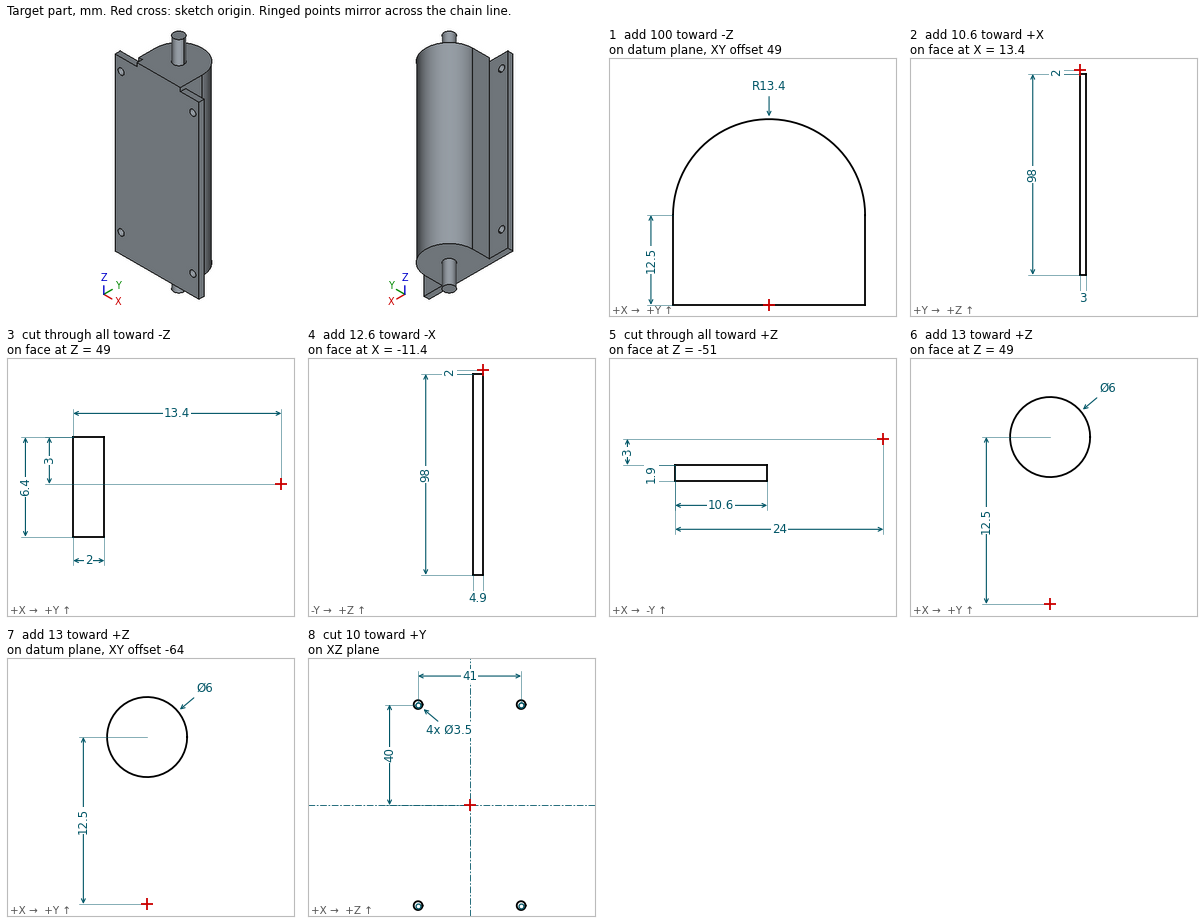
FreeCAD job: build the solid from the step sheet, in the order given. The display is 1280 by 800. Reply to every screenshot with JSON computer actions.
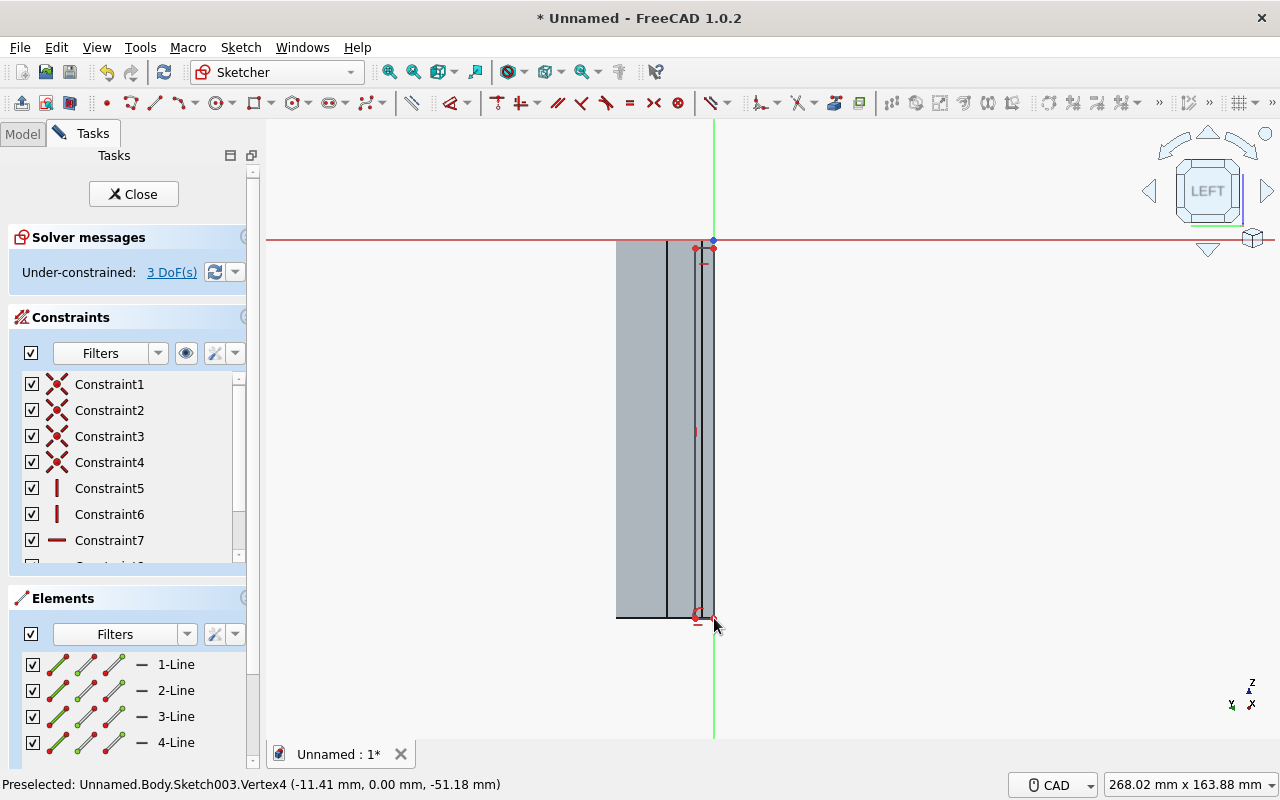
{"action": "left_click", "coordinate": [450, 104]}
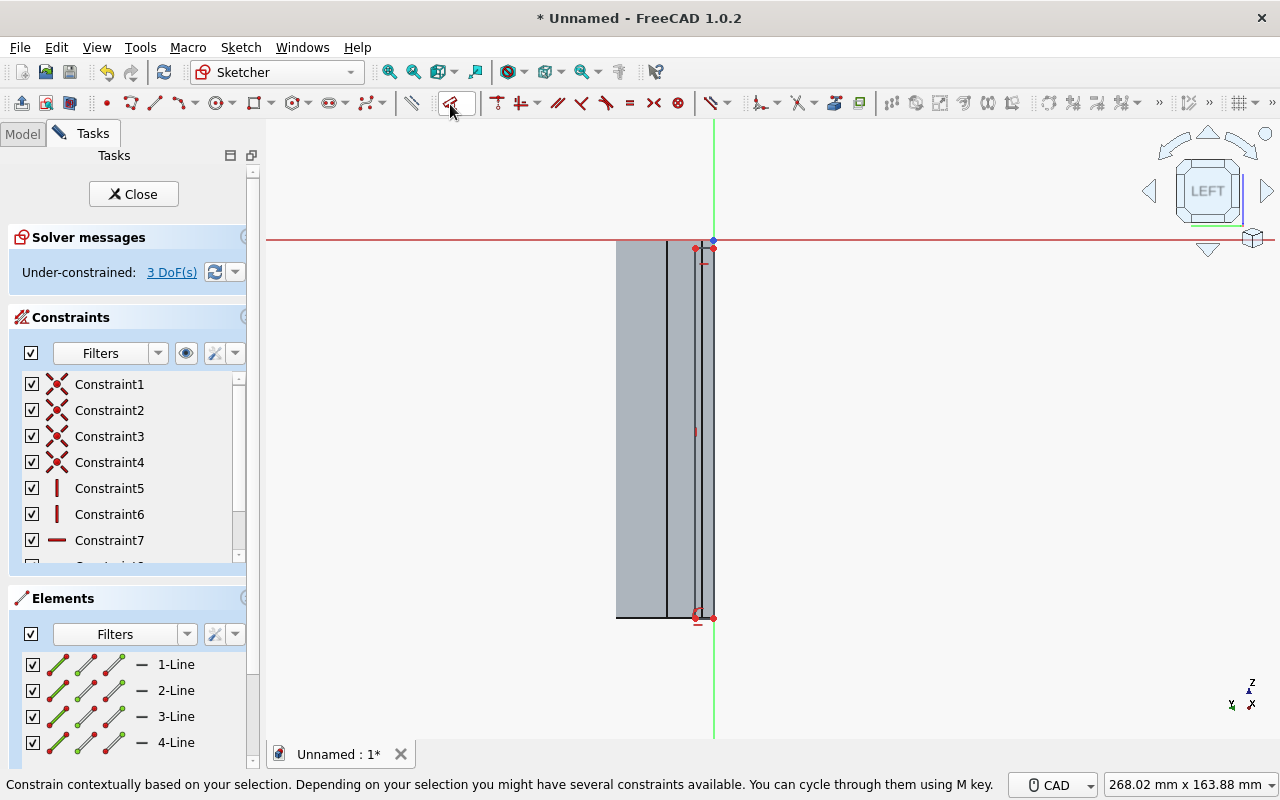
{"action": "left_click", "coordinate": [695, 359]}
{"action": "left_click", "coordinate": [661, 434]}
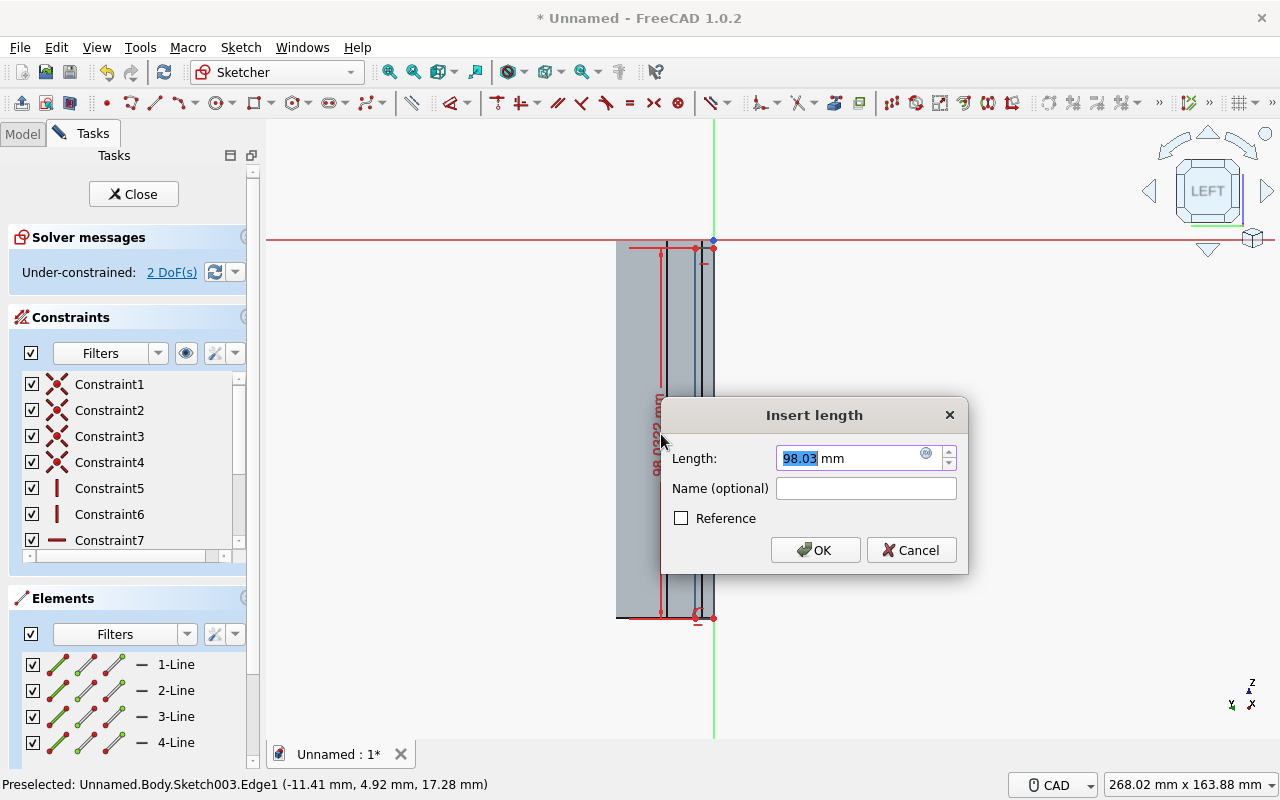
{"action": "type", "text": "98"}
{"action": "key", "text": "Return"}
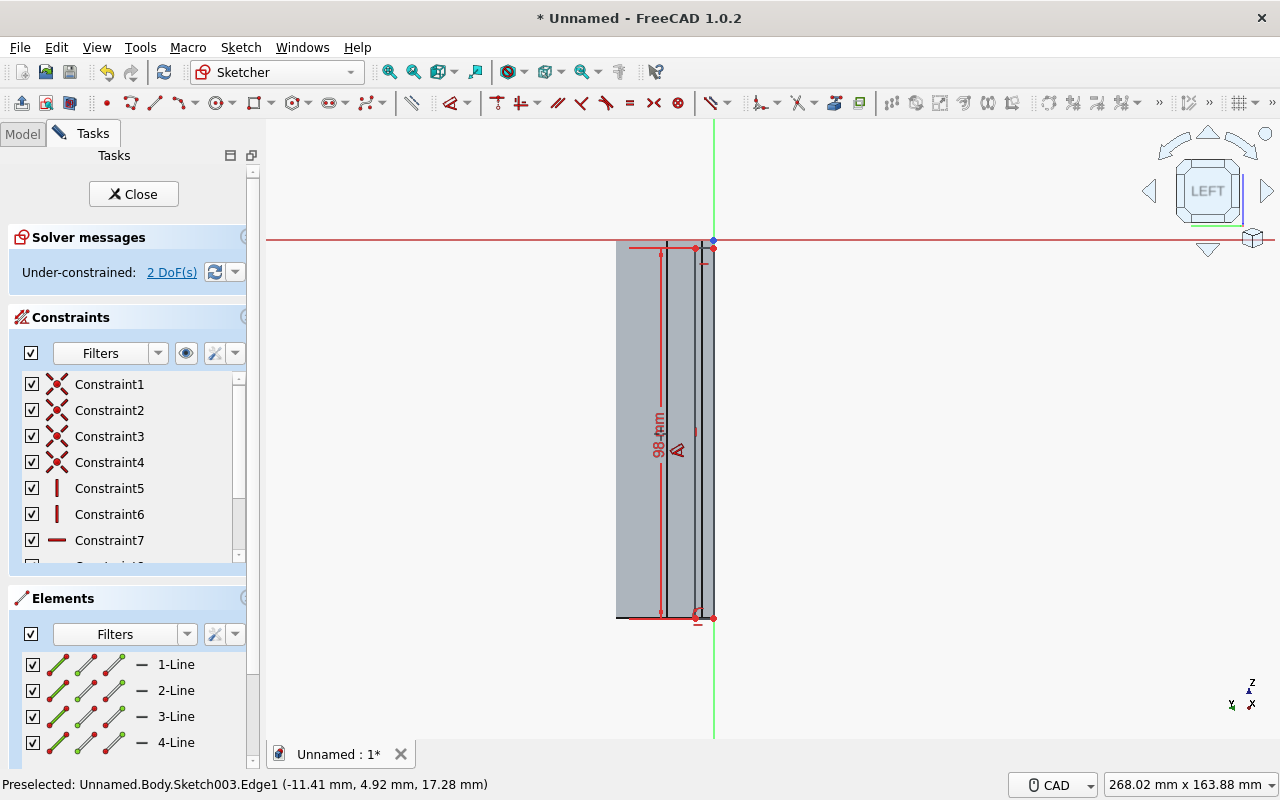
{"action": "scroll", "coordinate": [695, 248], "scroll_direction": "up", "scroll_amount": 9}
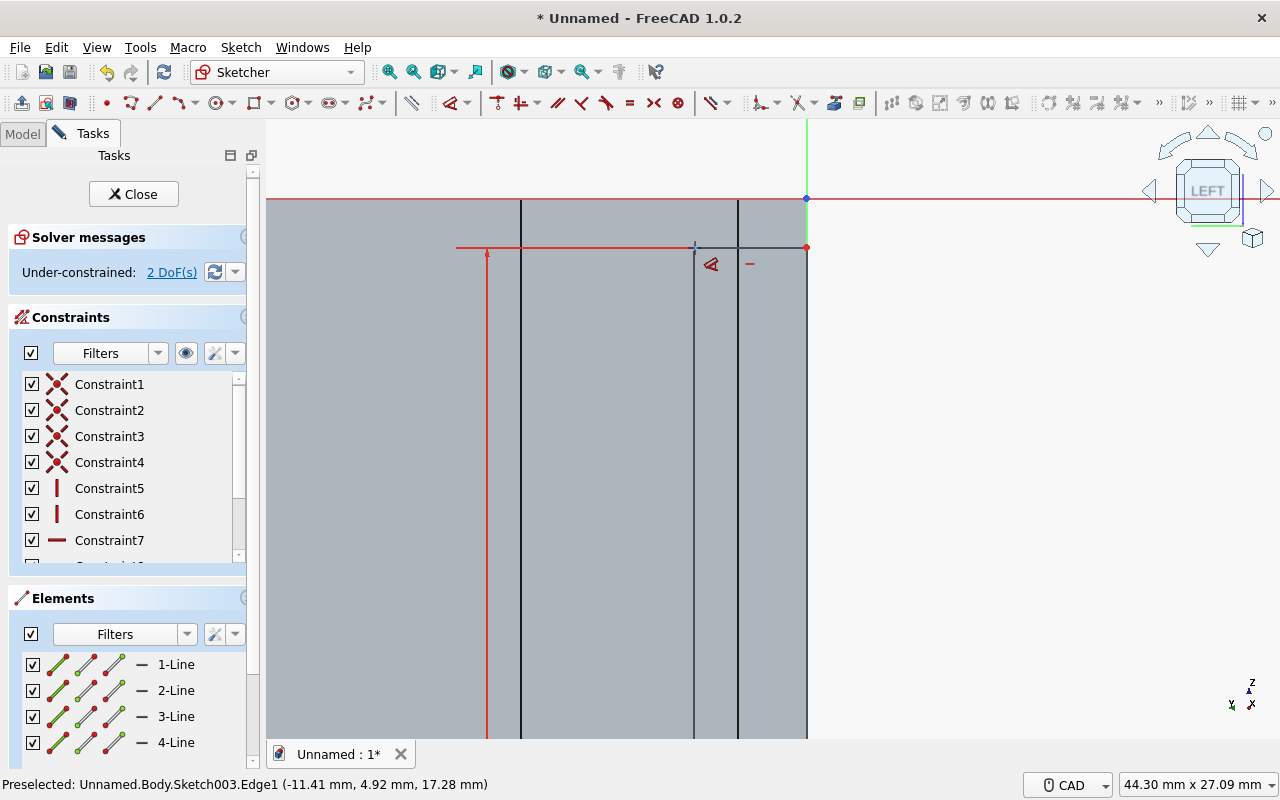
{"action": "left_click", "coordinate": [694, 248]}
{"action": "left_click", "coordinate": [660, 223]}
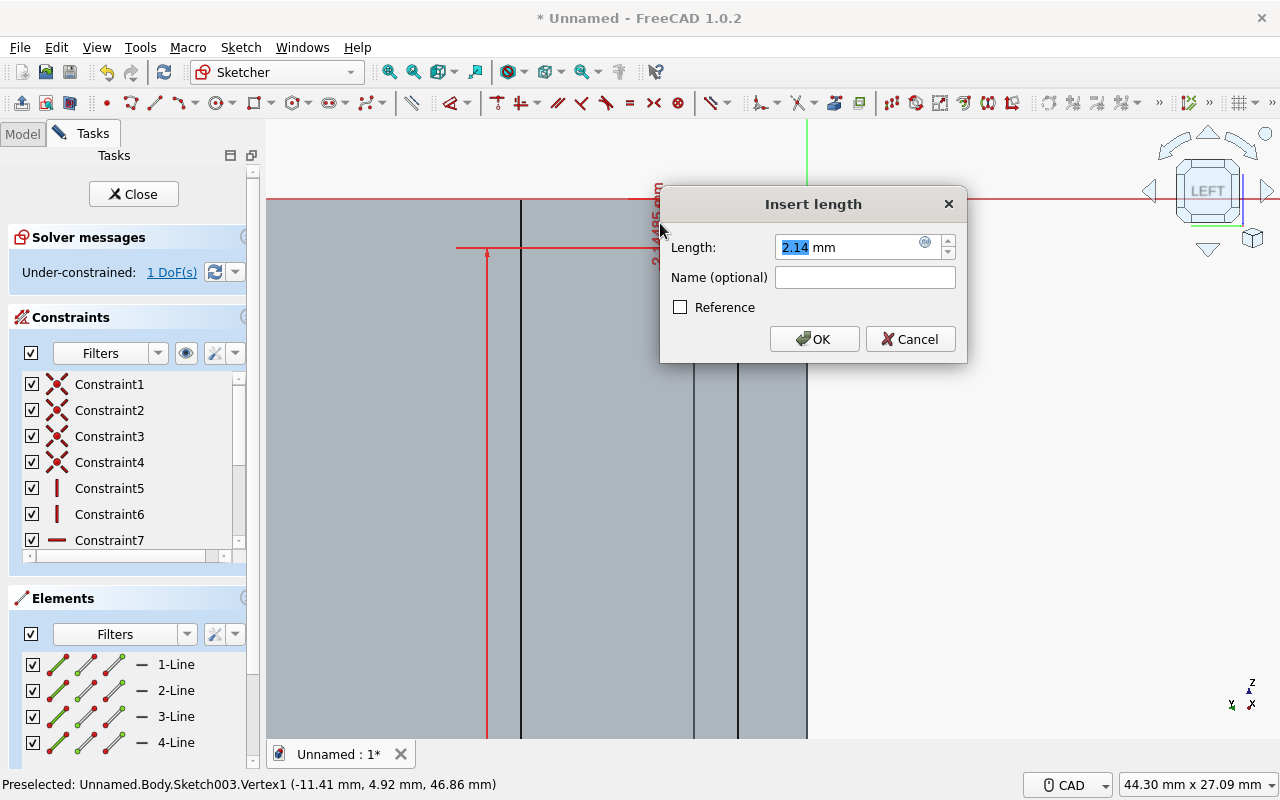
{"action": "type", "text": "2"}
{"action": "key", "text": "Return"}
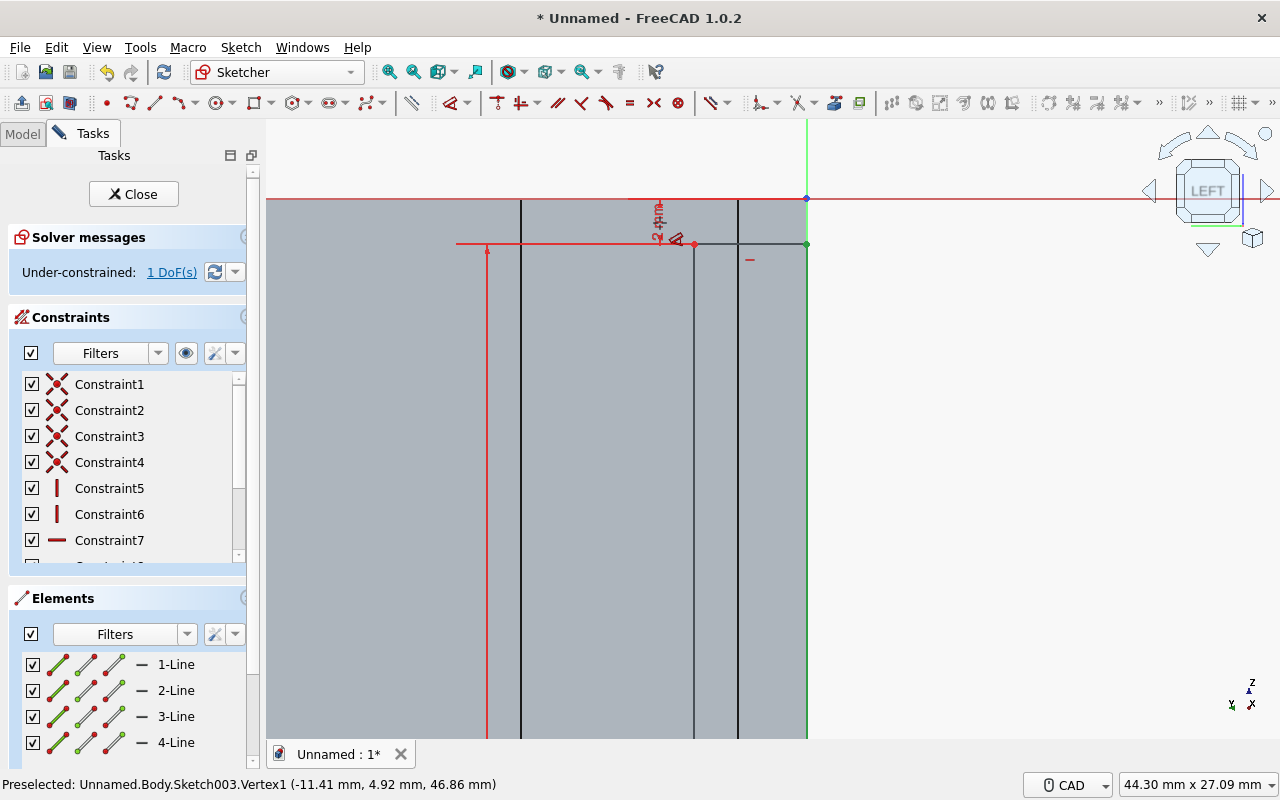
{"action": "scroll", "coordinate": [695, 248], "scroll_direction": "down", "scroll_amount": 9}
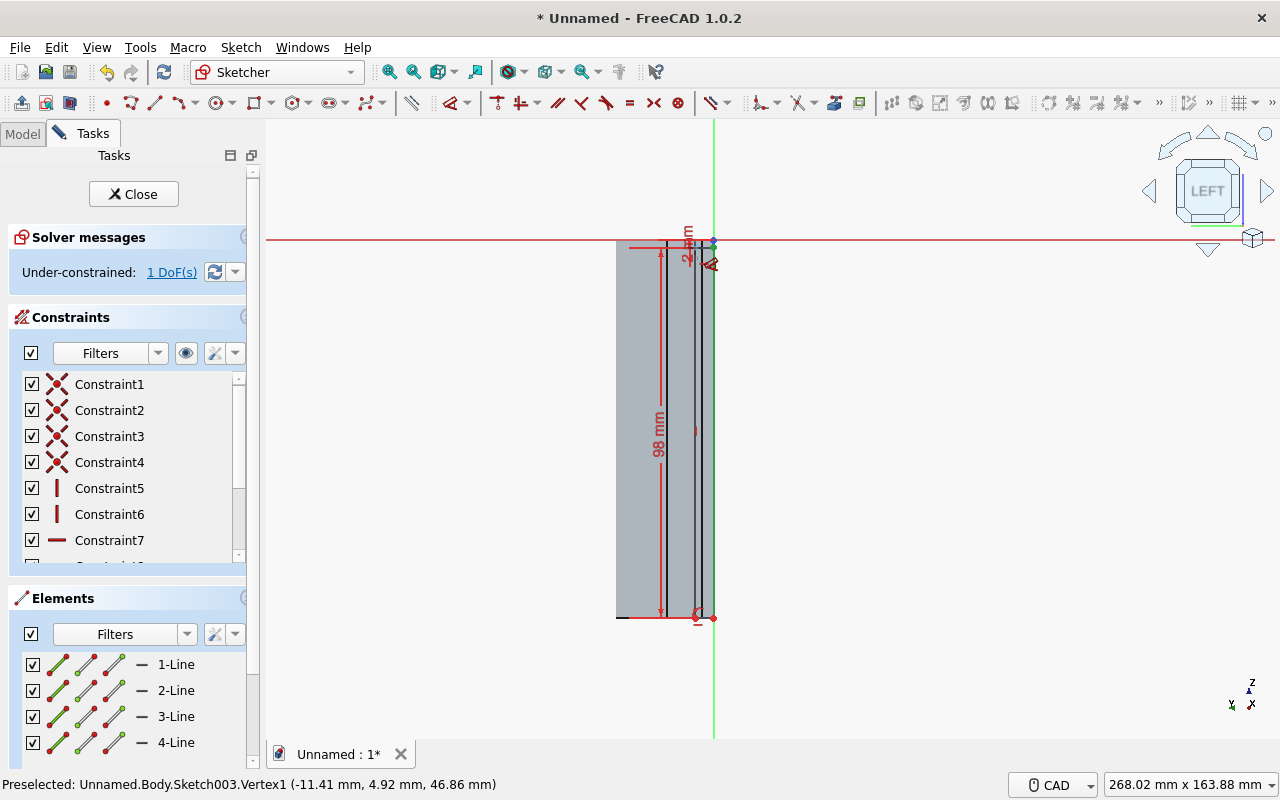
{"action": "scroll", "coordinate": [701, 618], "scroll_direction": "up", "scroll_amount": 5}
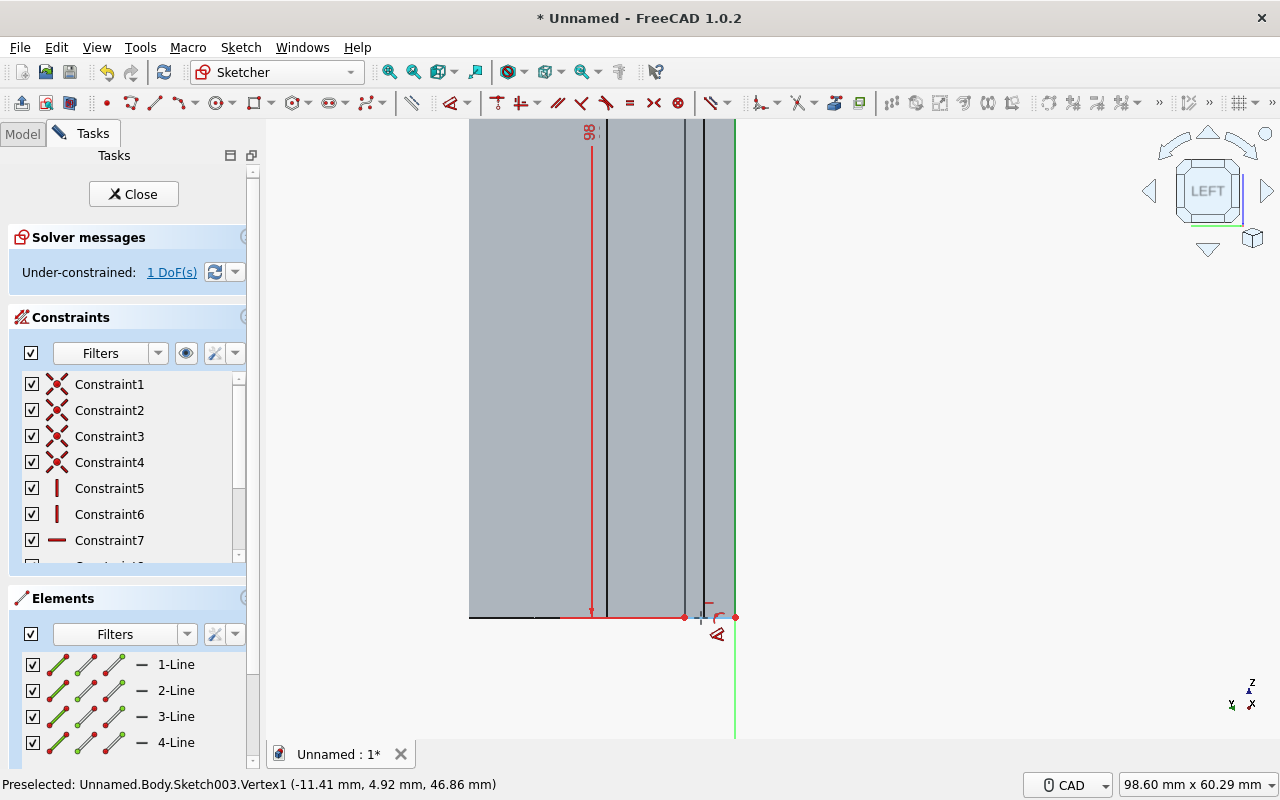
{"action": "left_click", "coordinate": [700, 618]}
{"action": "left_click", "coordinate": [710, 652]}